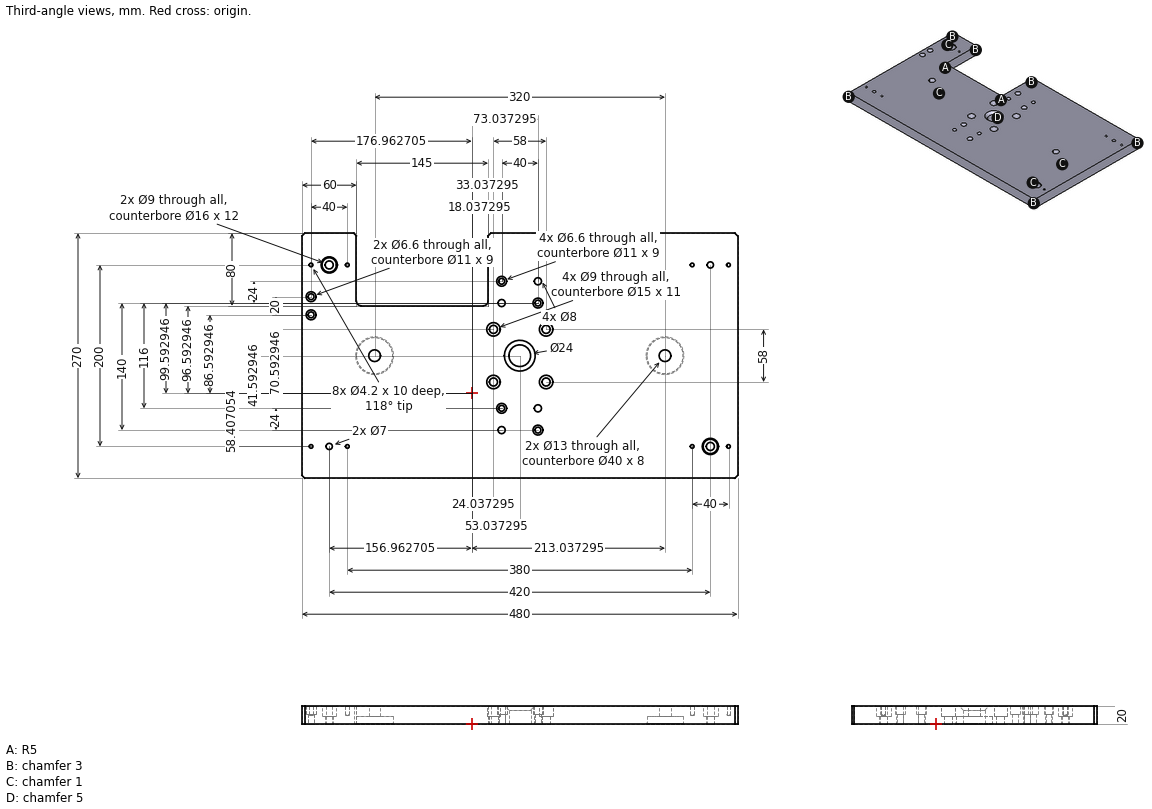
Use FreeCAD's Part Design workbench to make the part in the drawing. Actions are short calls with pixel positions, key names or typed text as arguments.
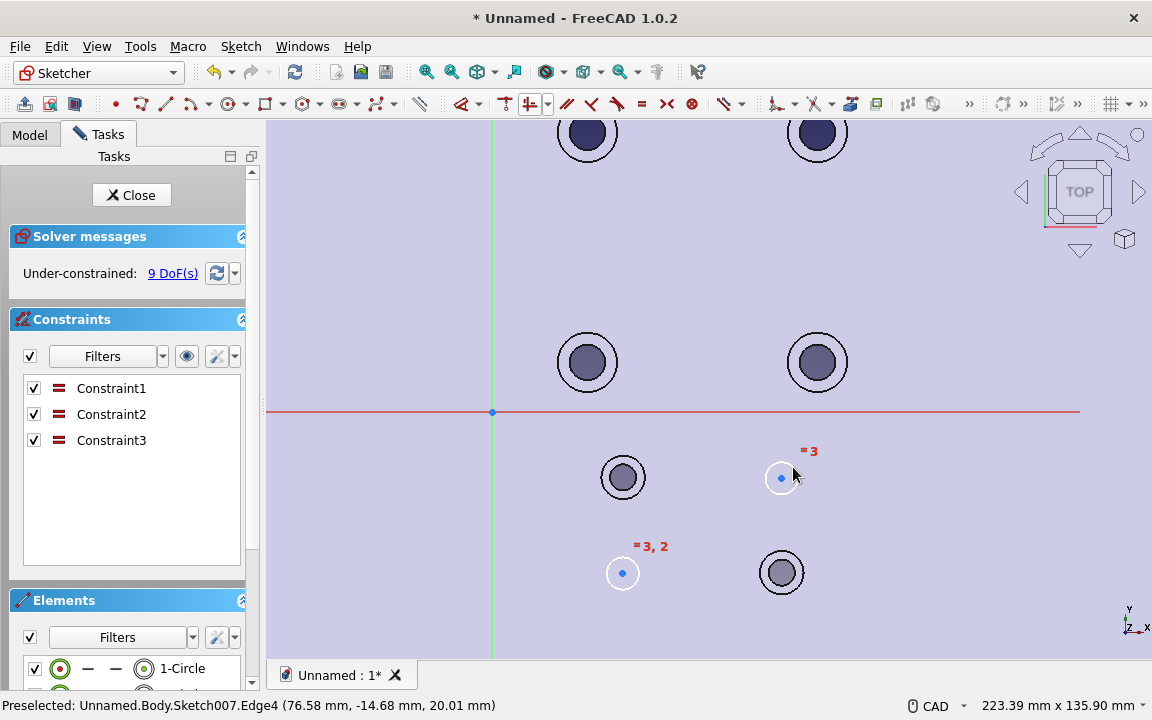
scroll(635, 562, down, 3)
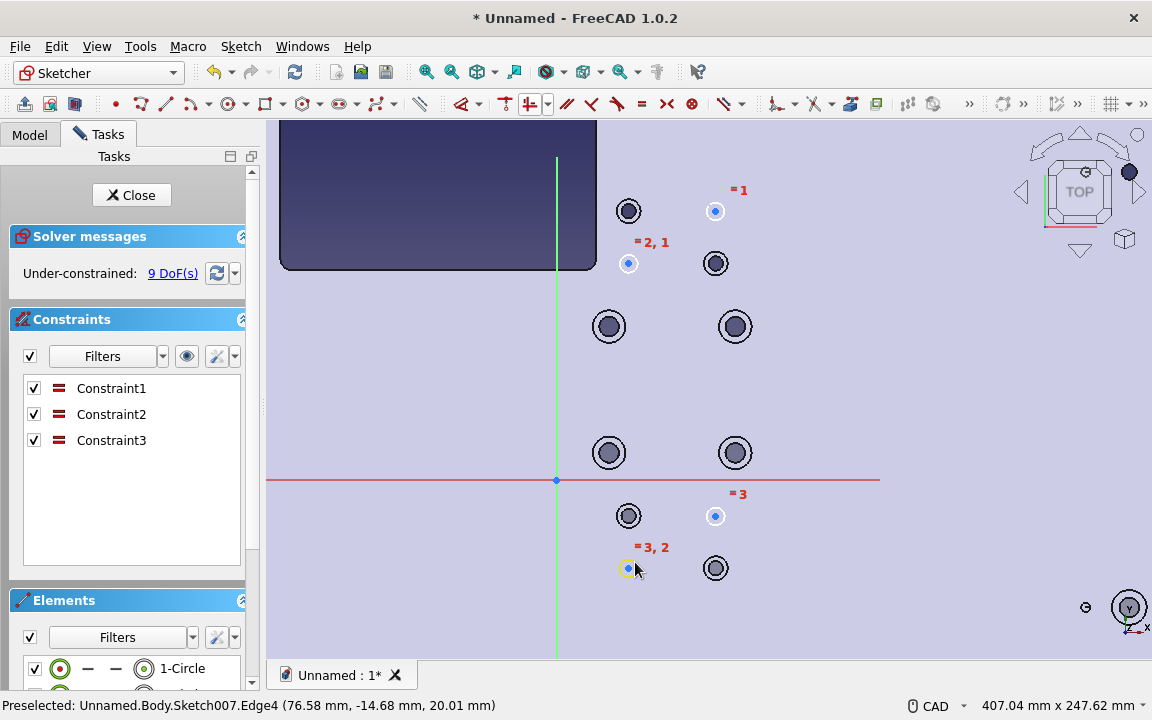
click(629, 264)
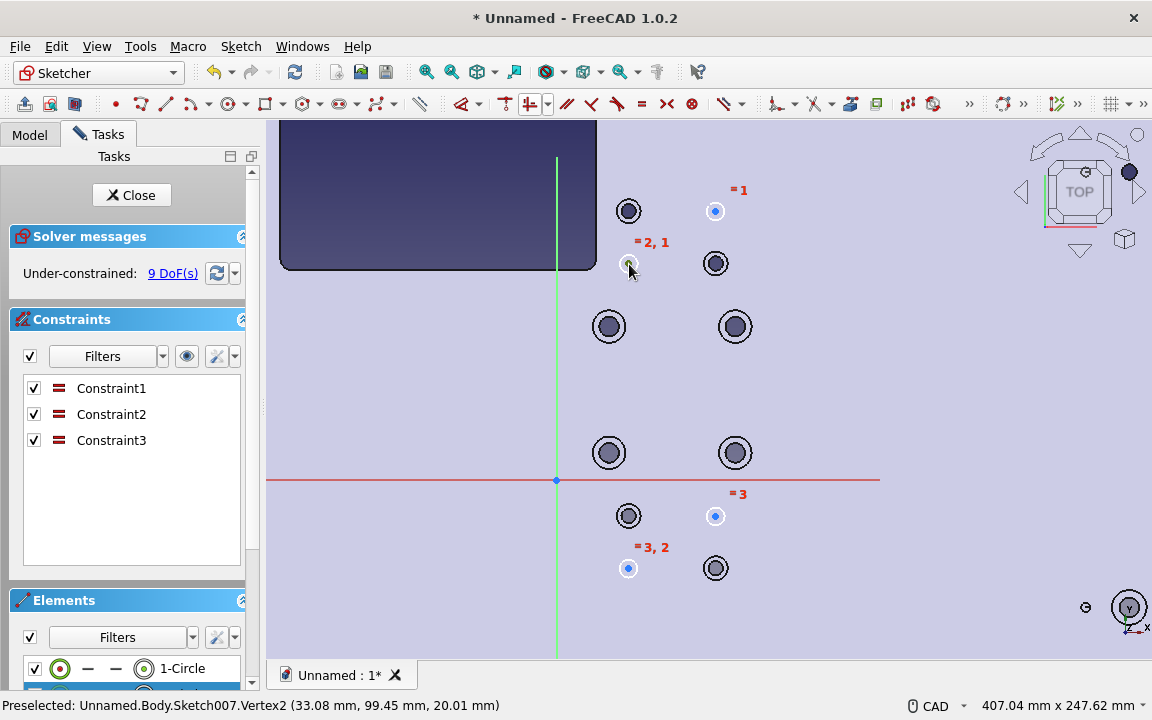
click(629, 569)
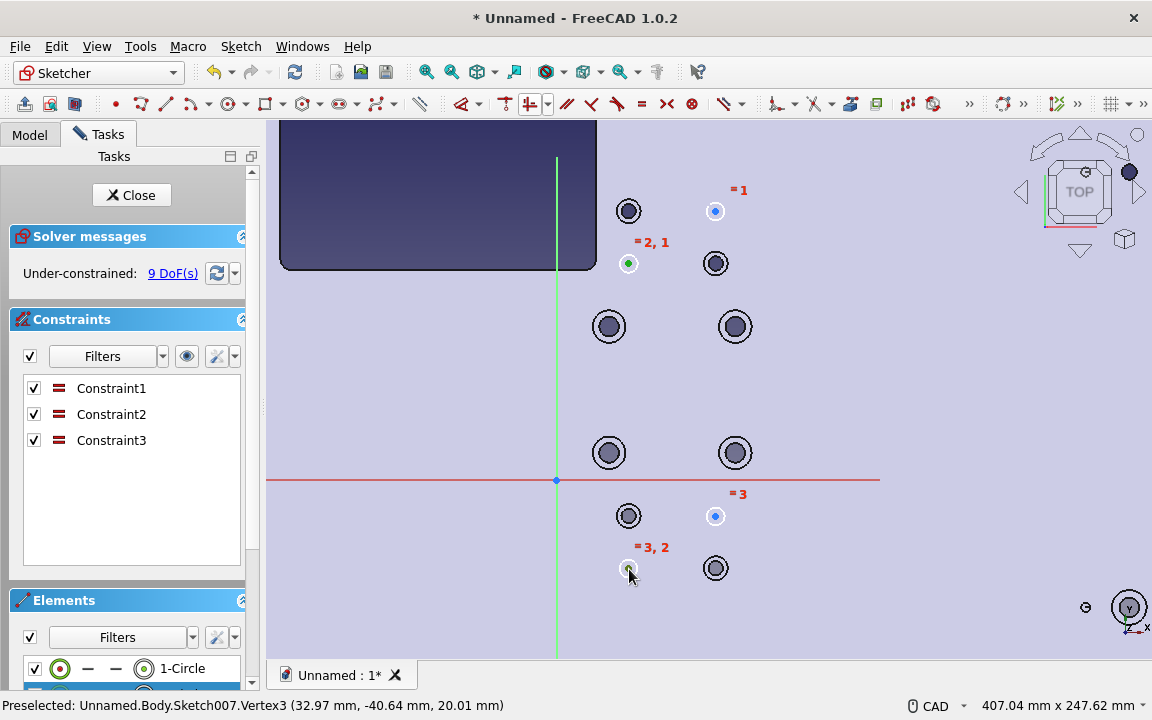
key(v)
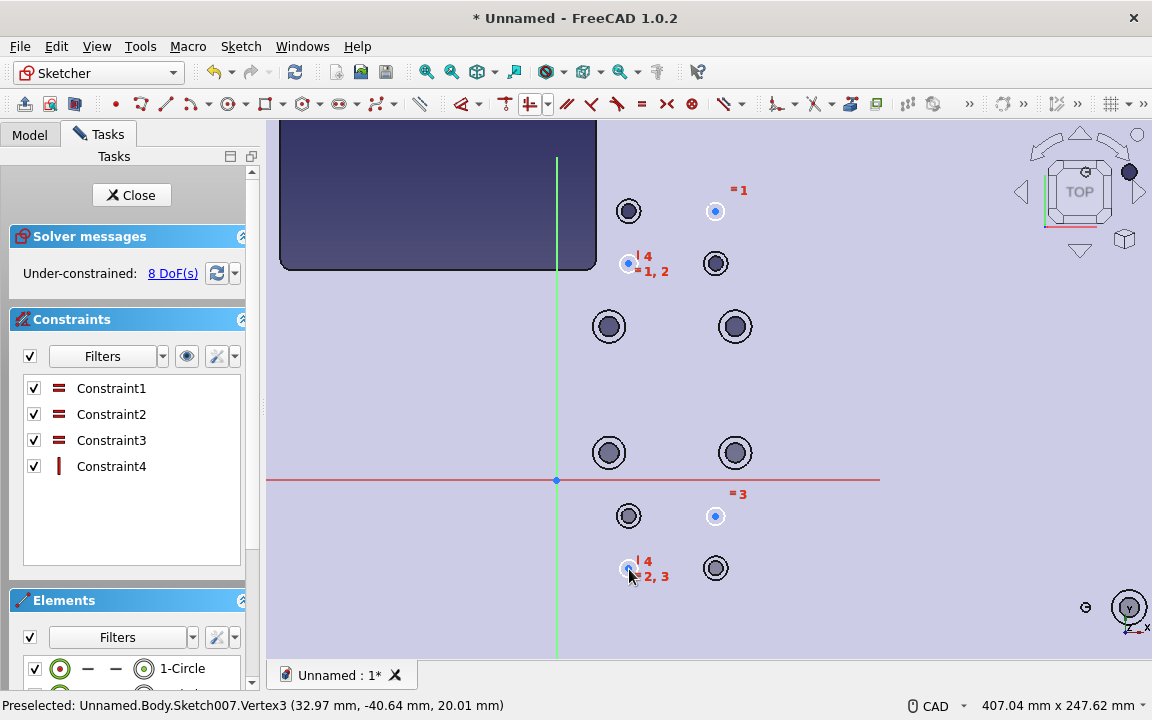
click(716, 212)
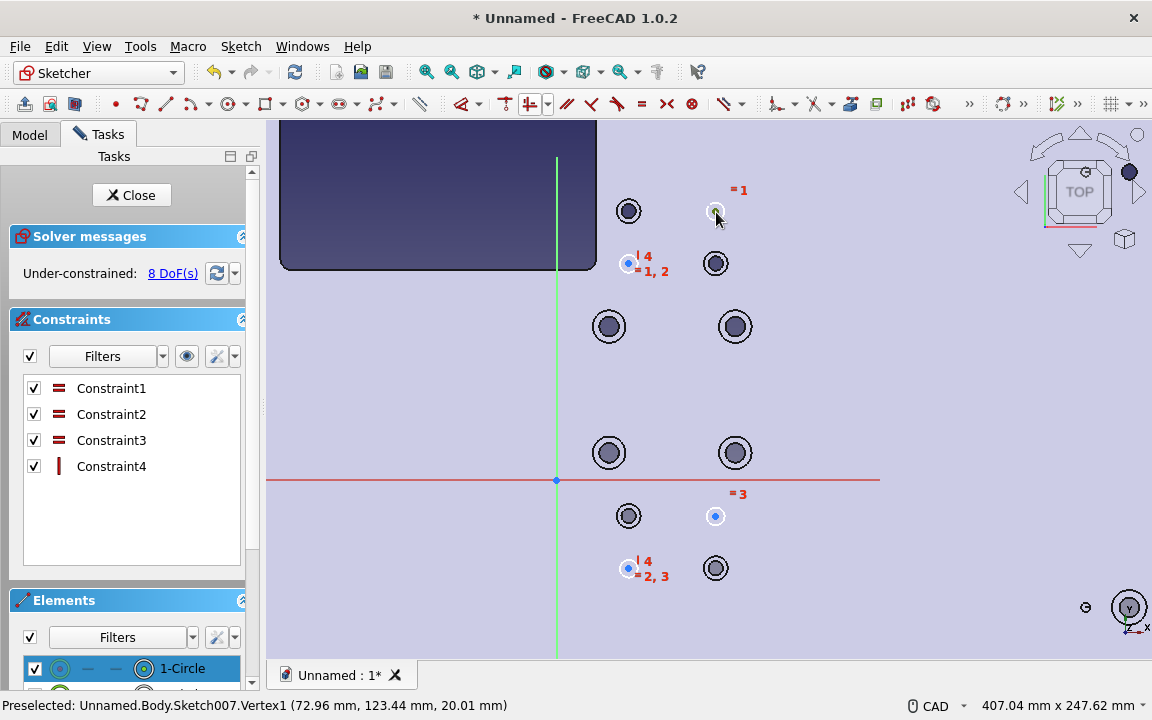
click(716, 516)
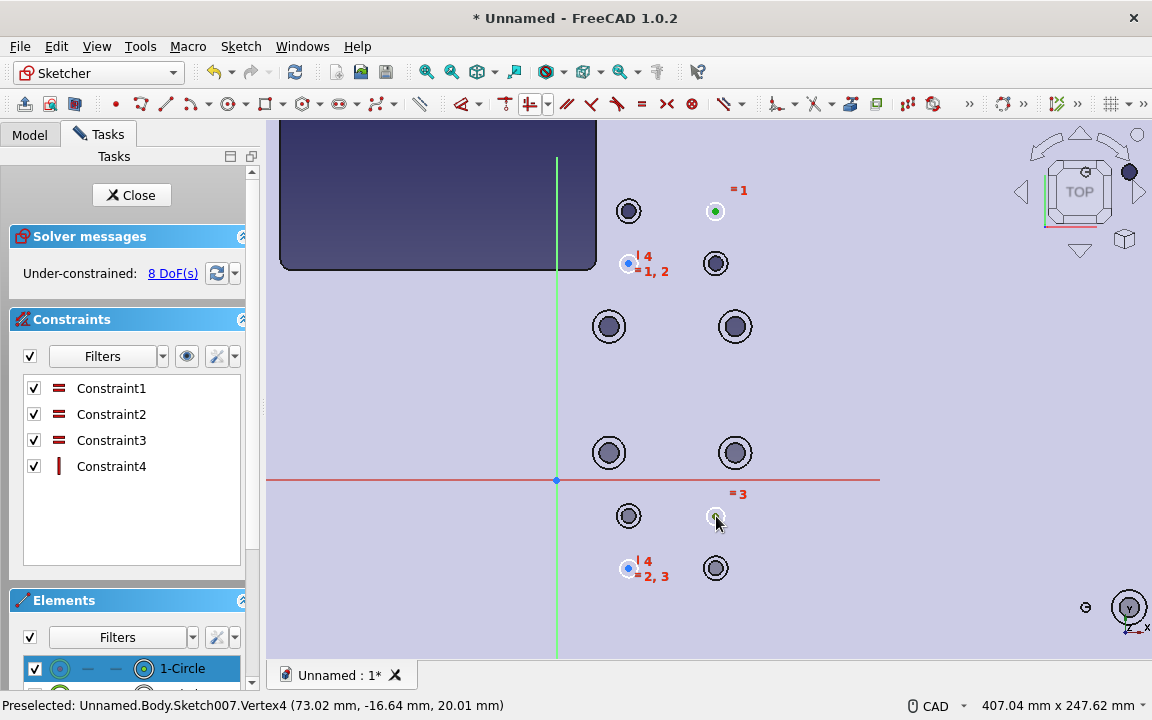
key(v)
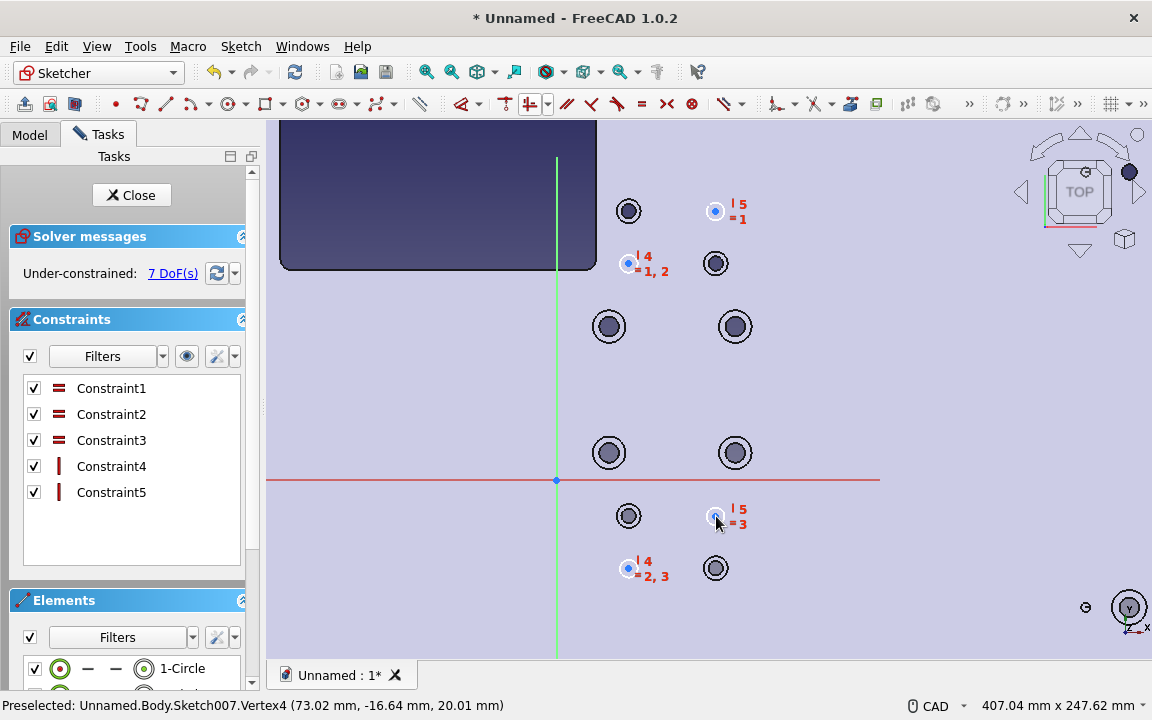
key(d)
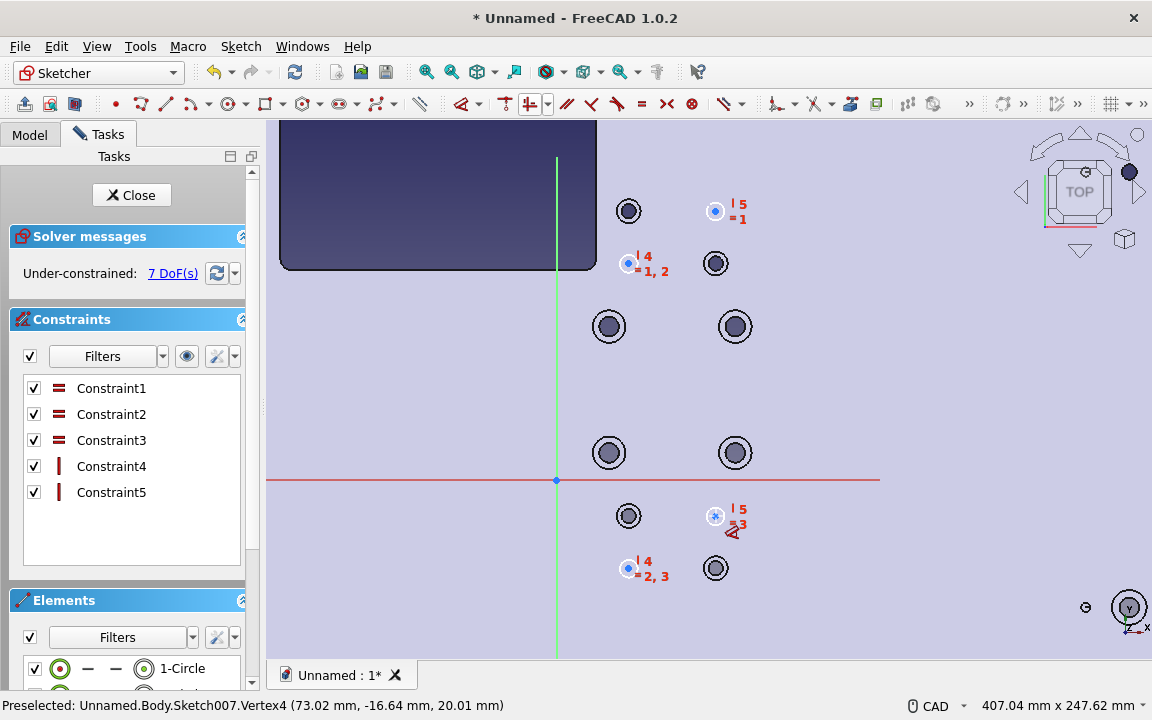
scroll(722, 205, up, 5)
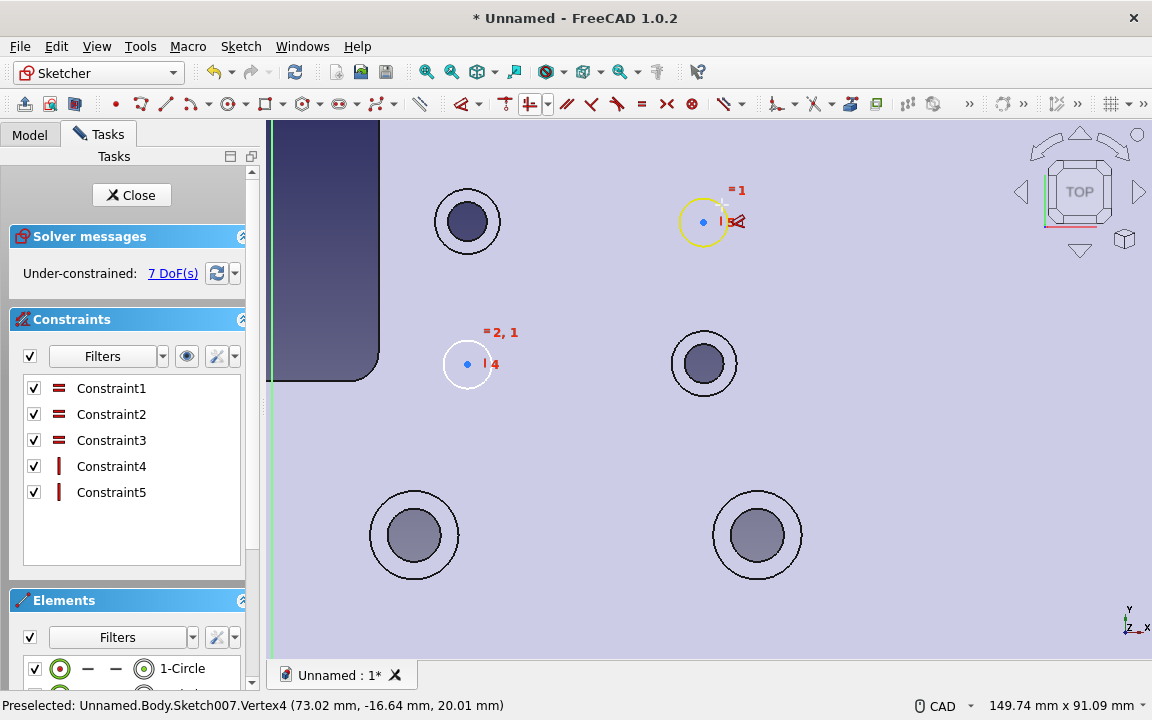
click(721, 205)
click(743, 182)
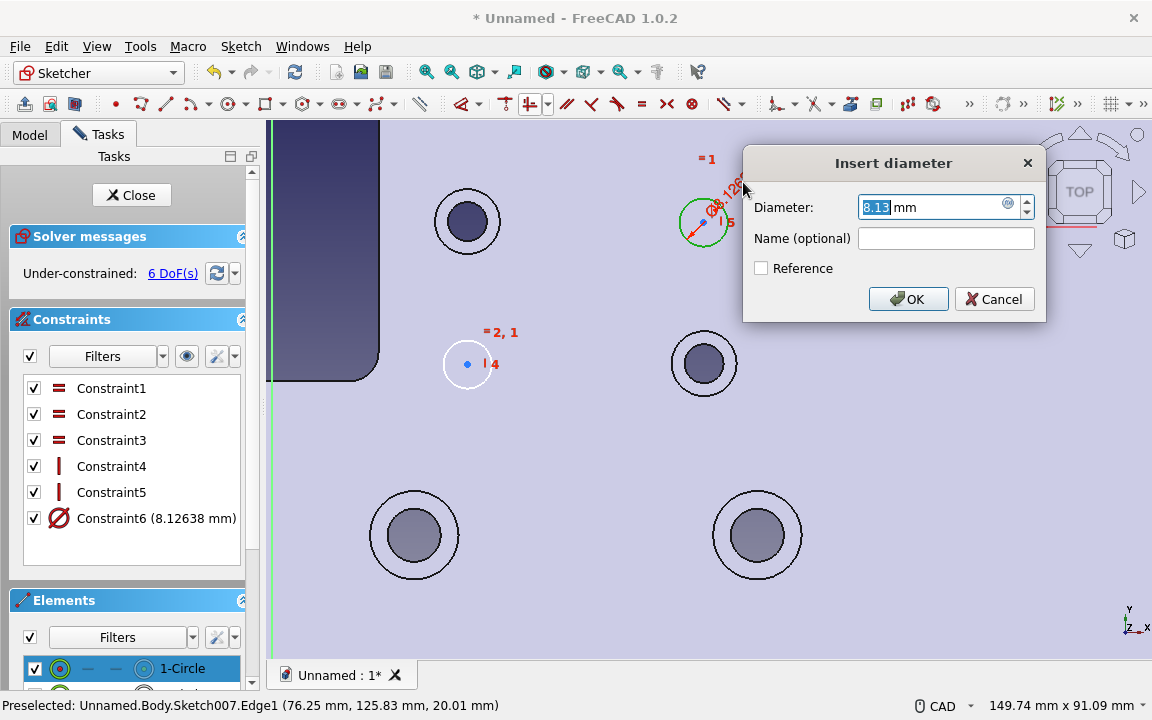
text(8)
key(Return)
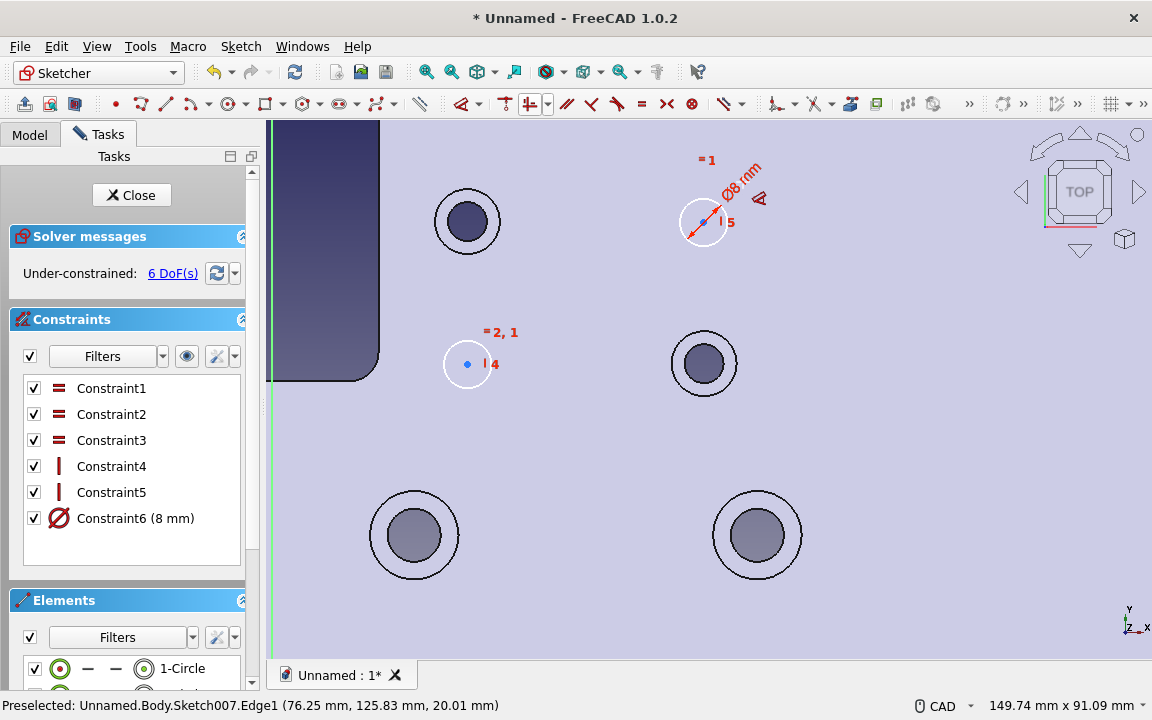
click(704, 223)